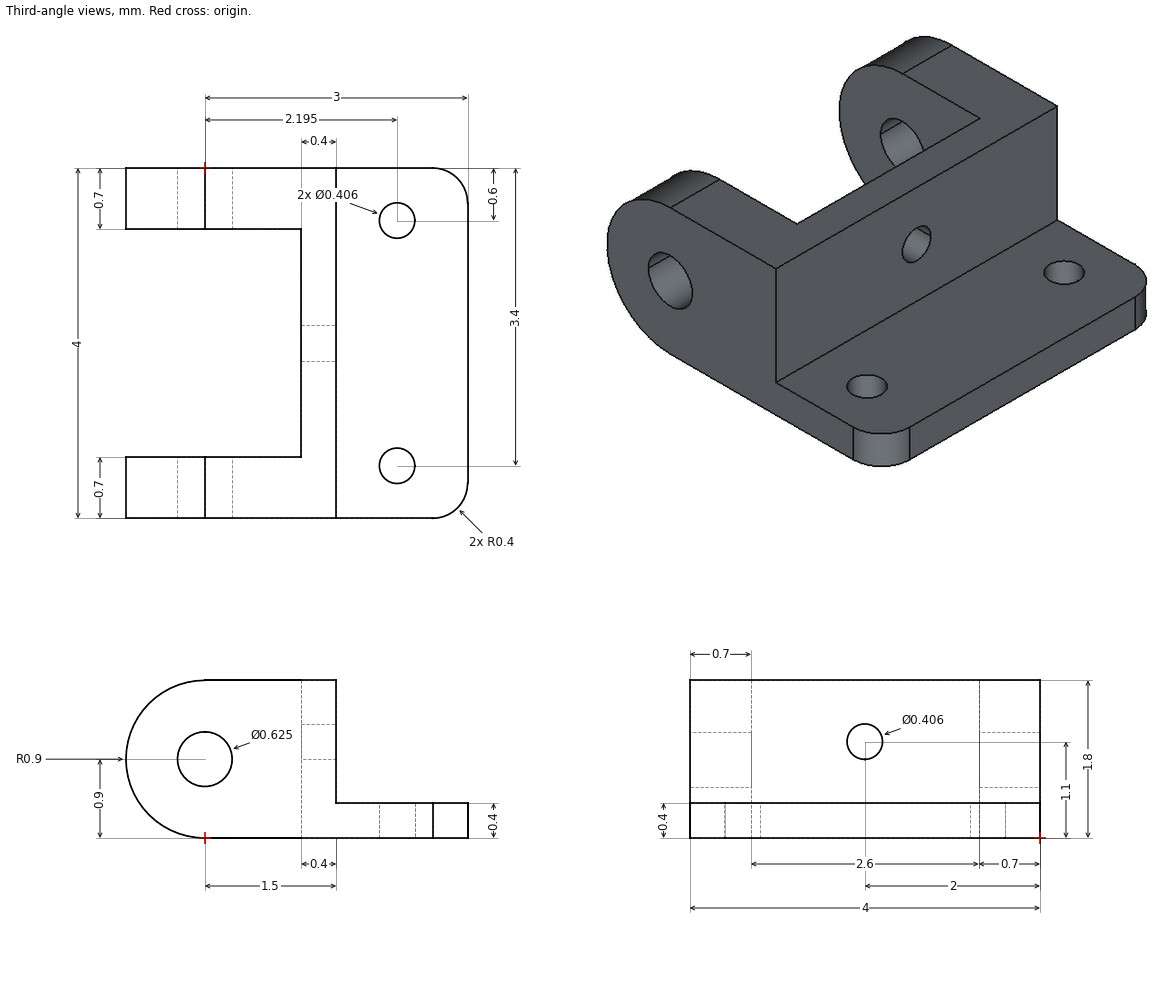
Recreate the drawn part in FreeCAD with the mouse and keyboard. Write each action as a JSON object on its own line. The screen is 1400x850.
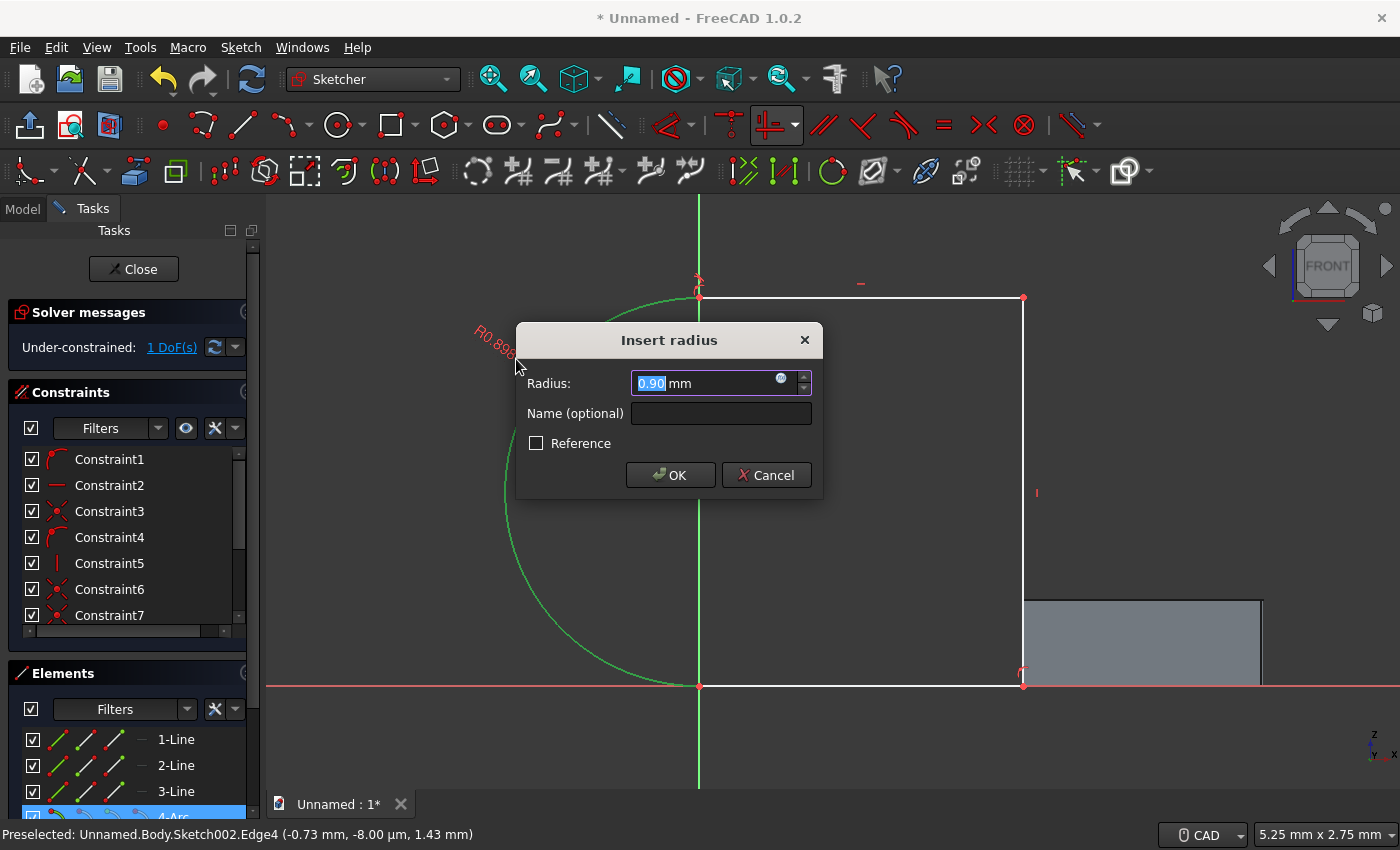
{"action": "type", "text": "0.9"}
{"action": "key", "text": "Return"}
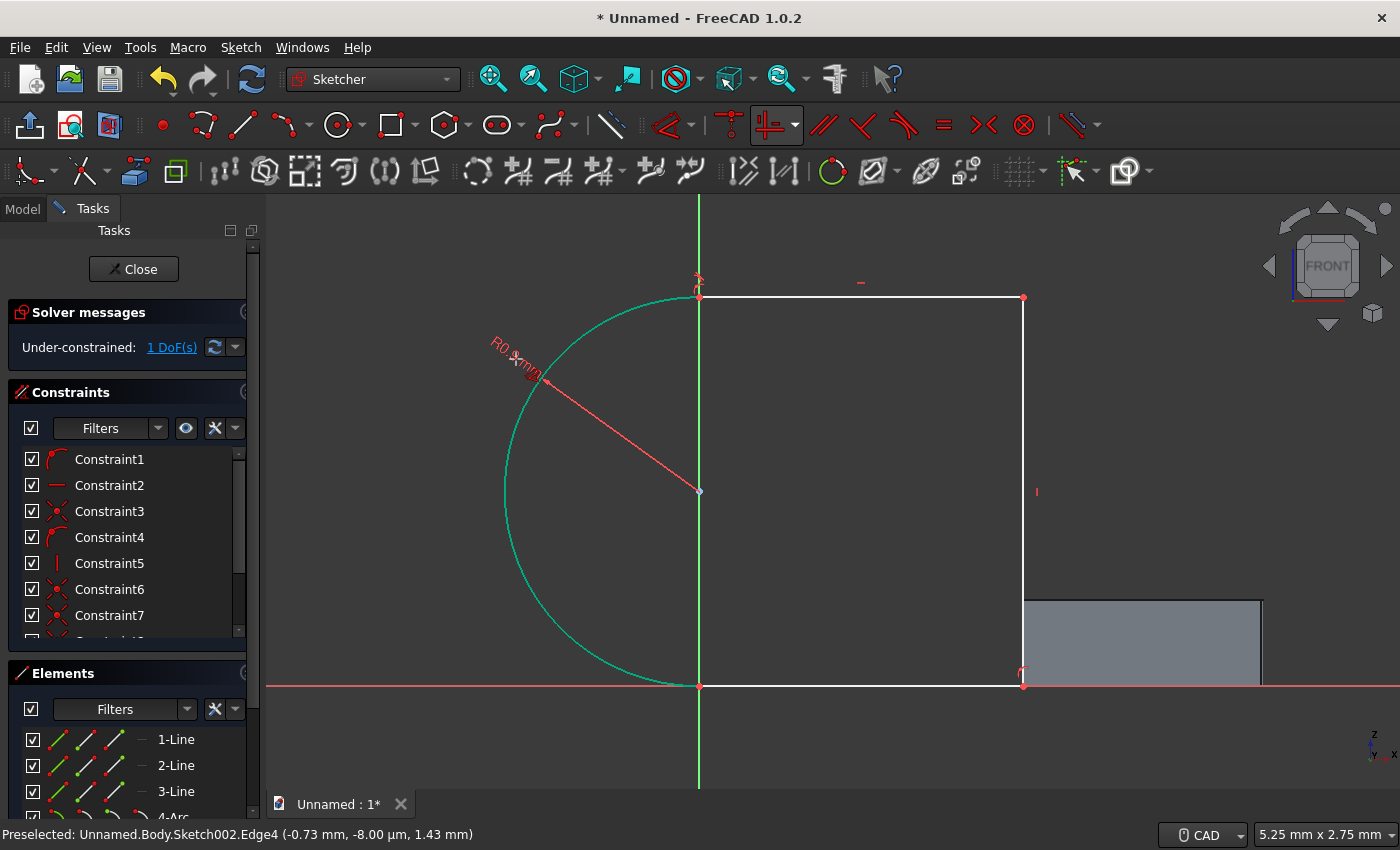
{"action": "left_click", "coordinate": [796, 297]}
{"action": "left_click", "coordinate": [861, 263]}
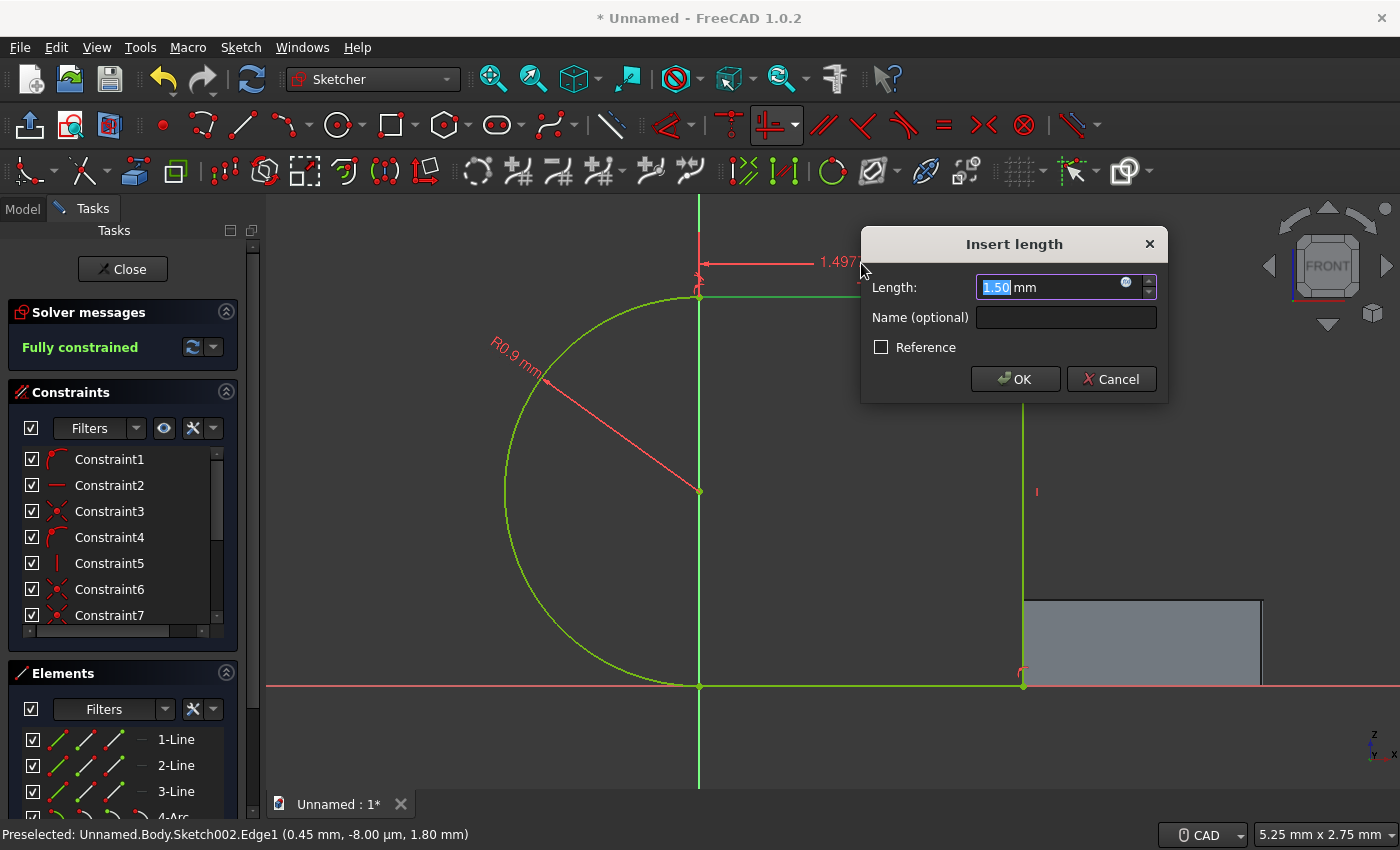
{"action": "type", "text": "1.5"}
{"action": "key", "text": "Return"}
{"action": "key", "text": "Escape"}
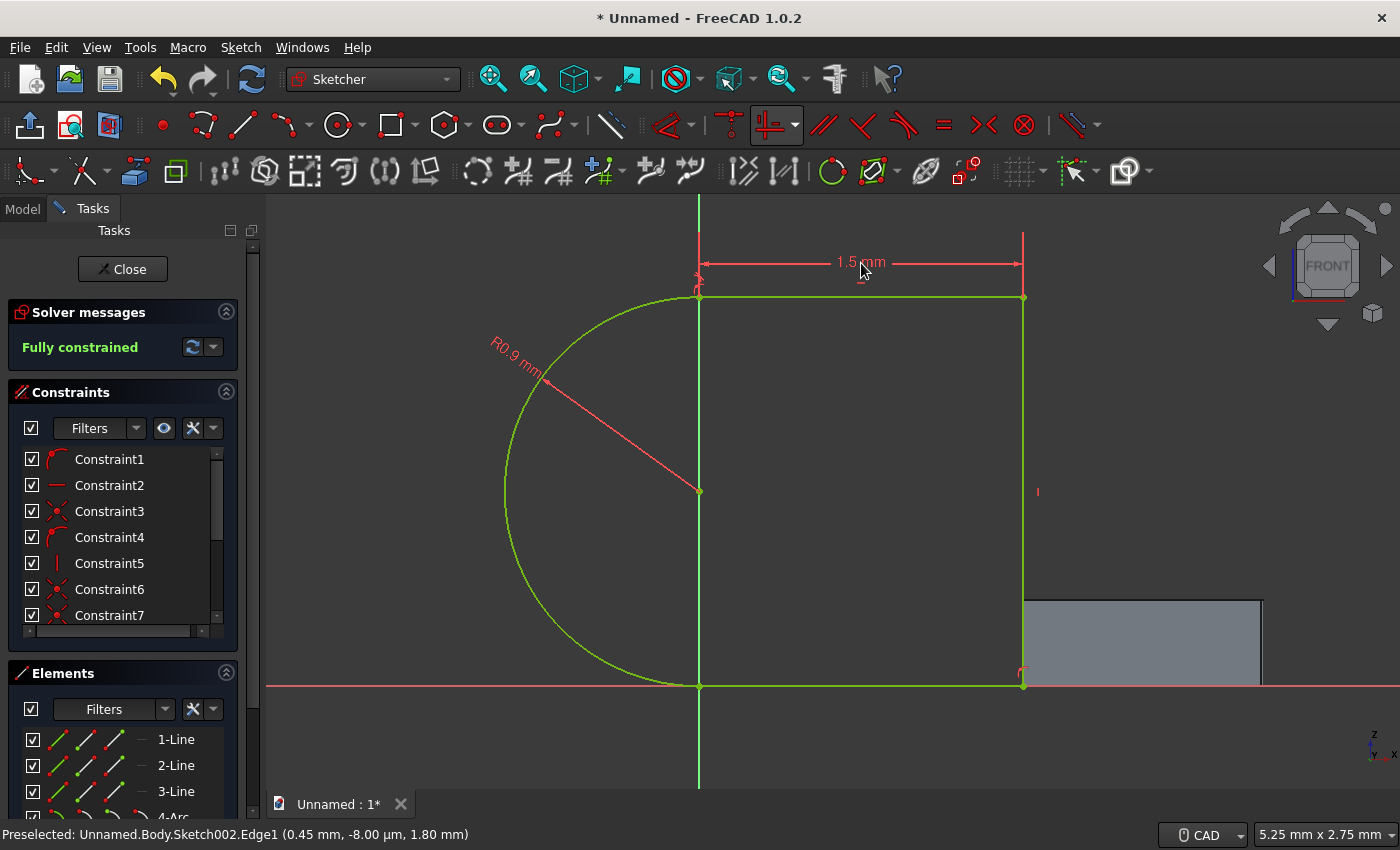
{"action": "left_click", "coordinate": [123, 269]}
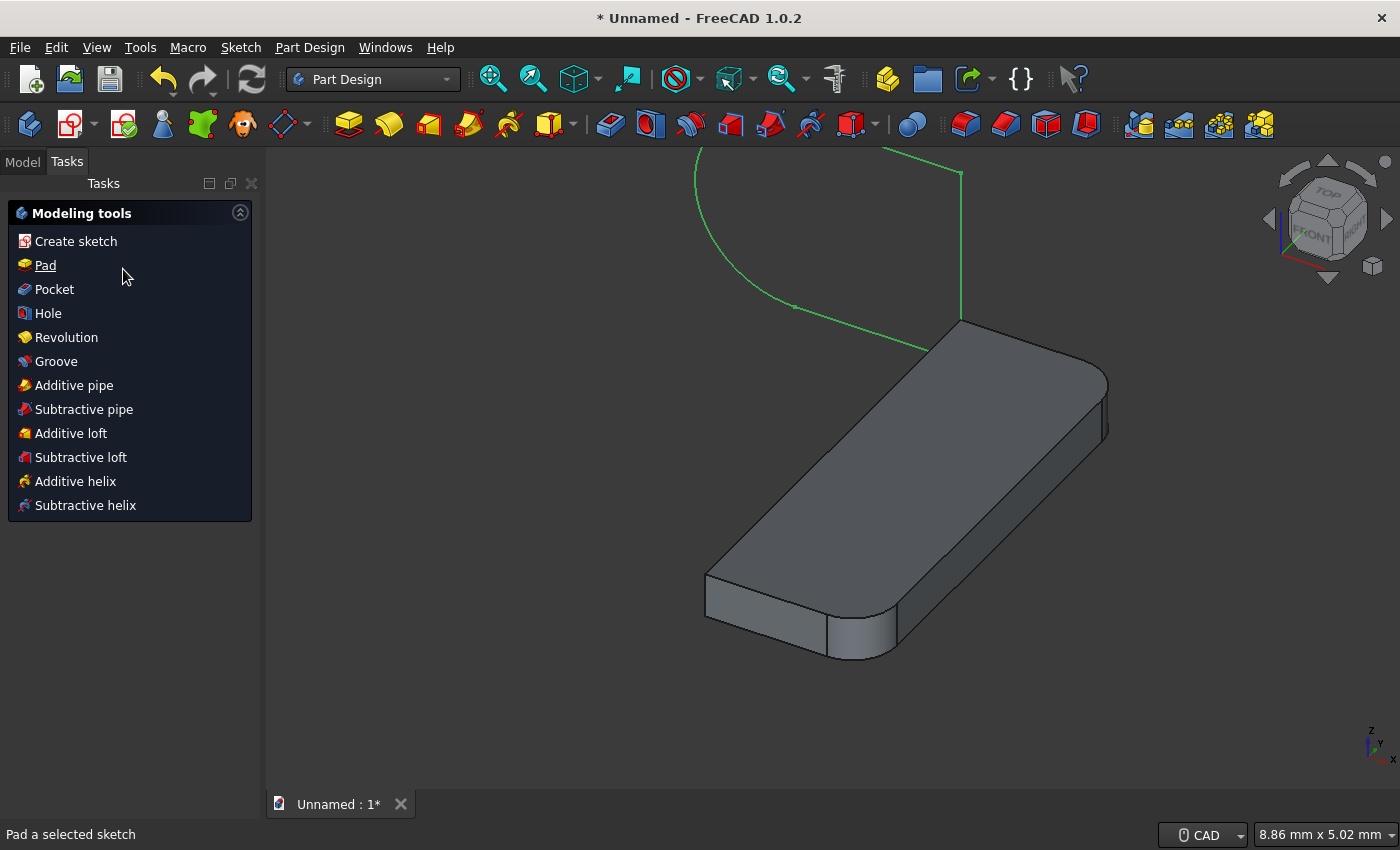
{"action": "left_click", "coordinate": [350, 124]}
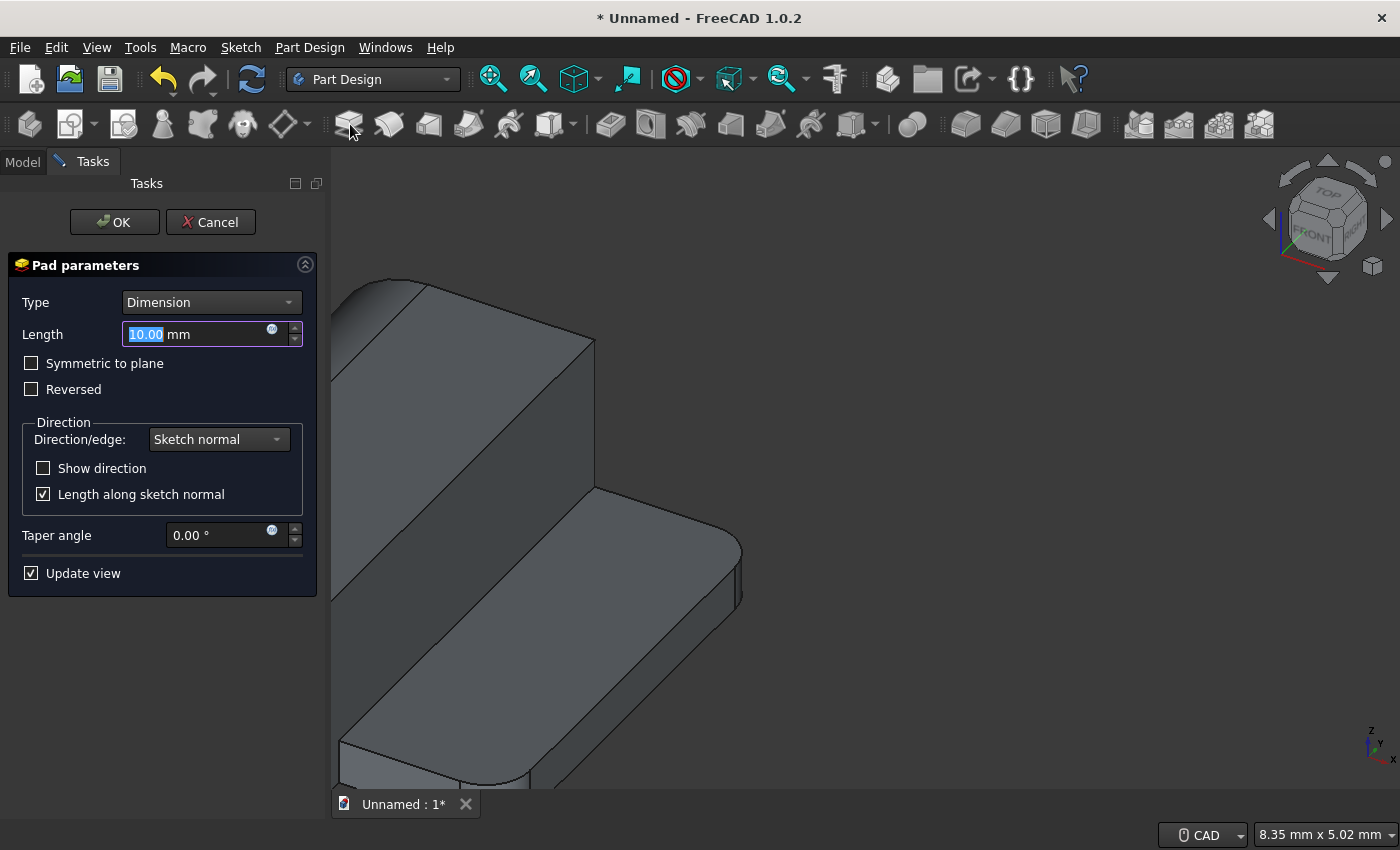
{"action": "type", "text": "0.7"}
{"action": "key", "text": "Tab"}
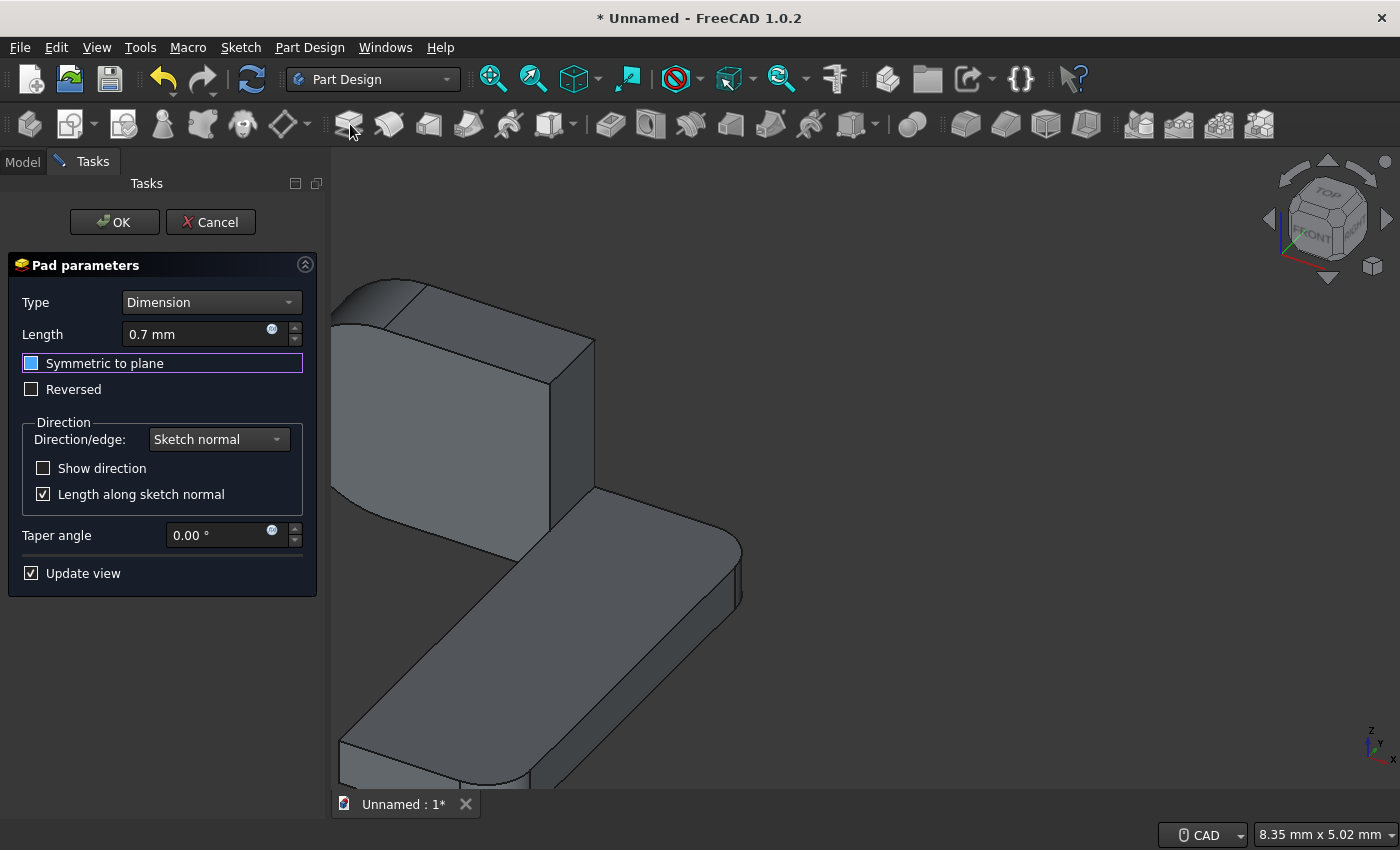
{"action": "left_click", "coordinate": [115, 222]}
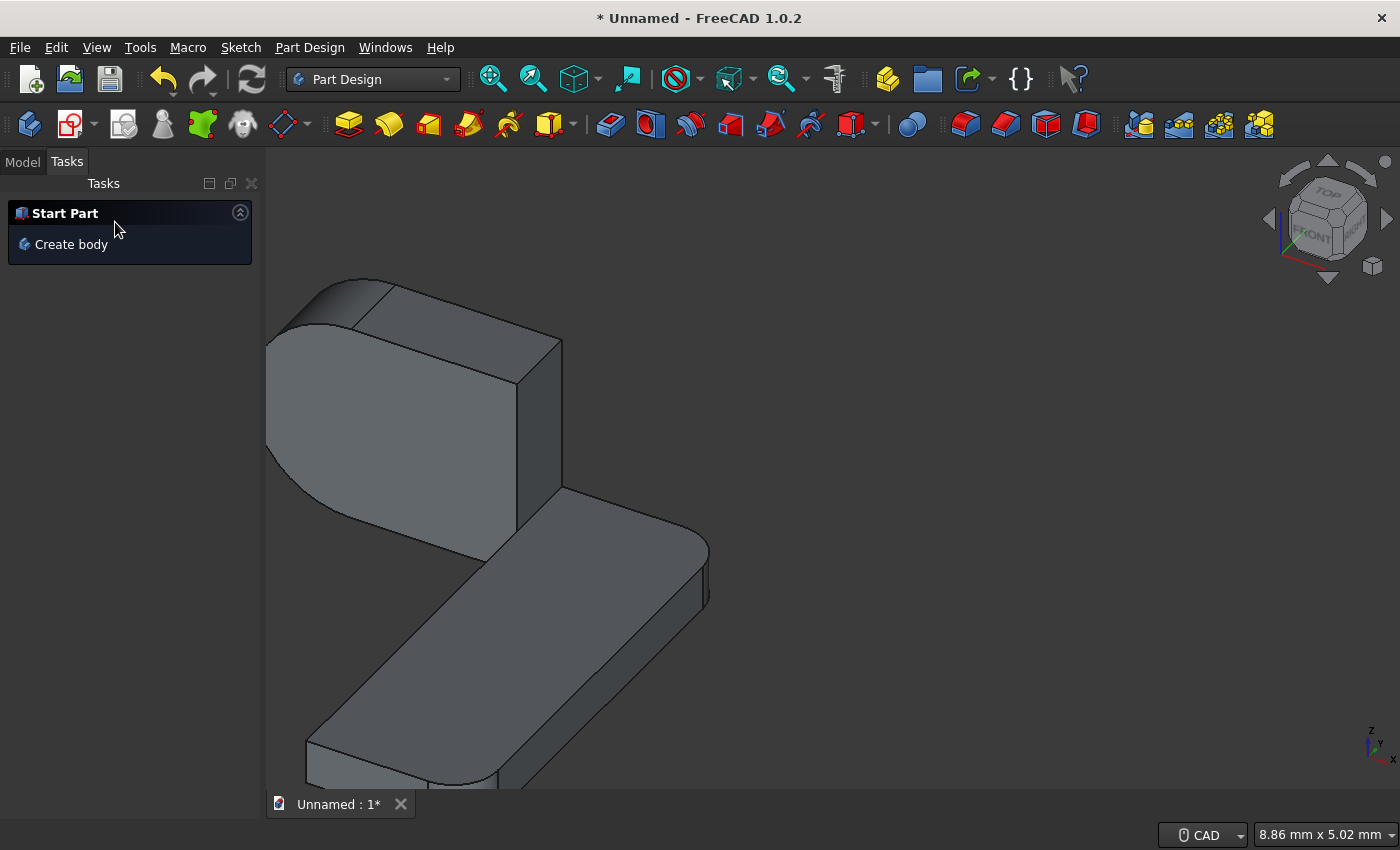
{"action": "left_click", "coordinate": [494, 80]}